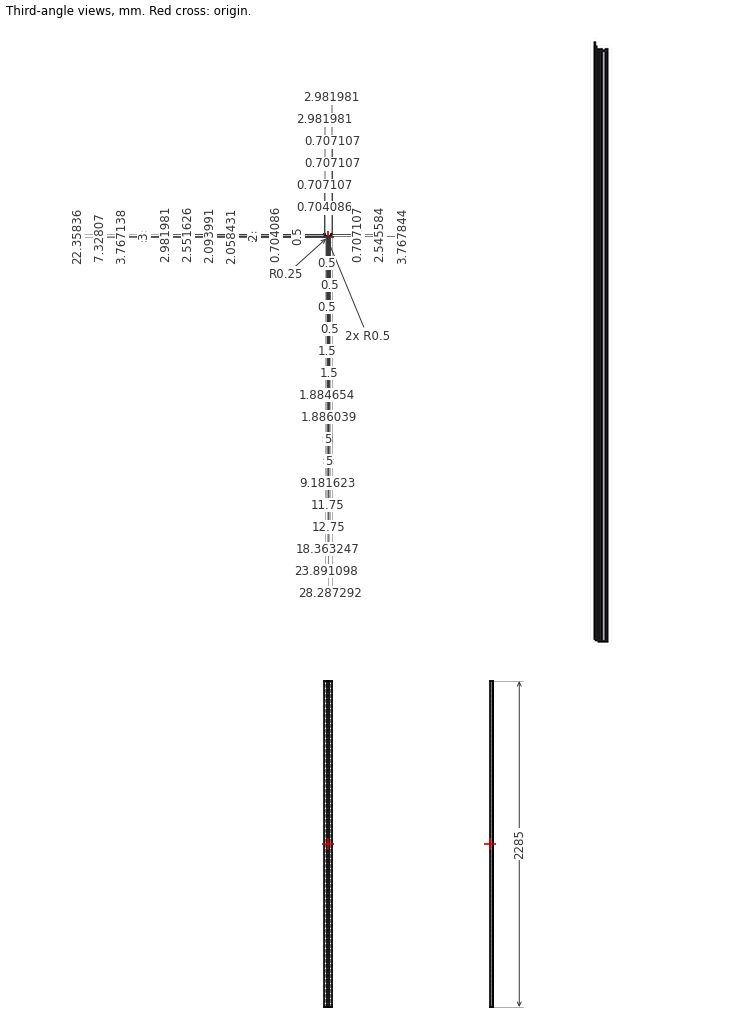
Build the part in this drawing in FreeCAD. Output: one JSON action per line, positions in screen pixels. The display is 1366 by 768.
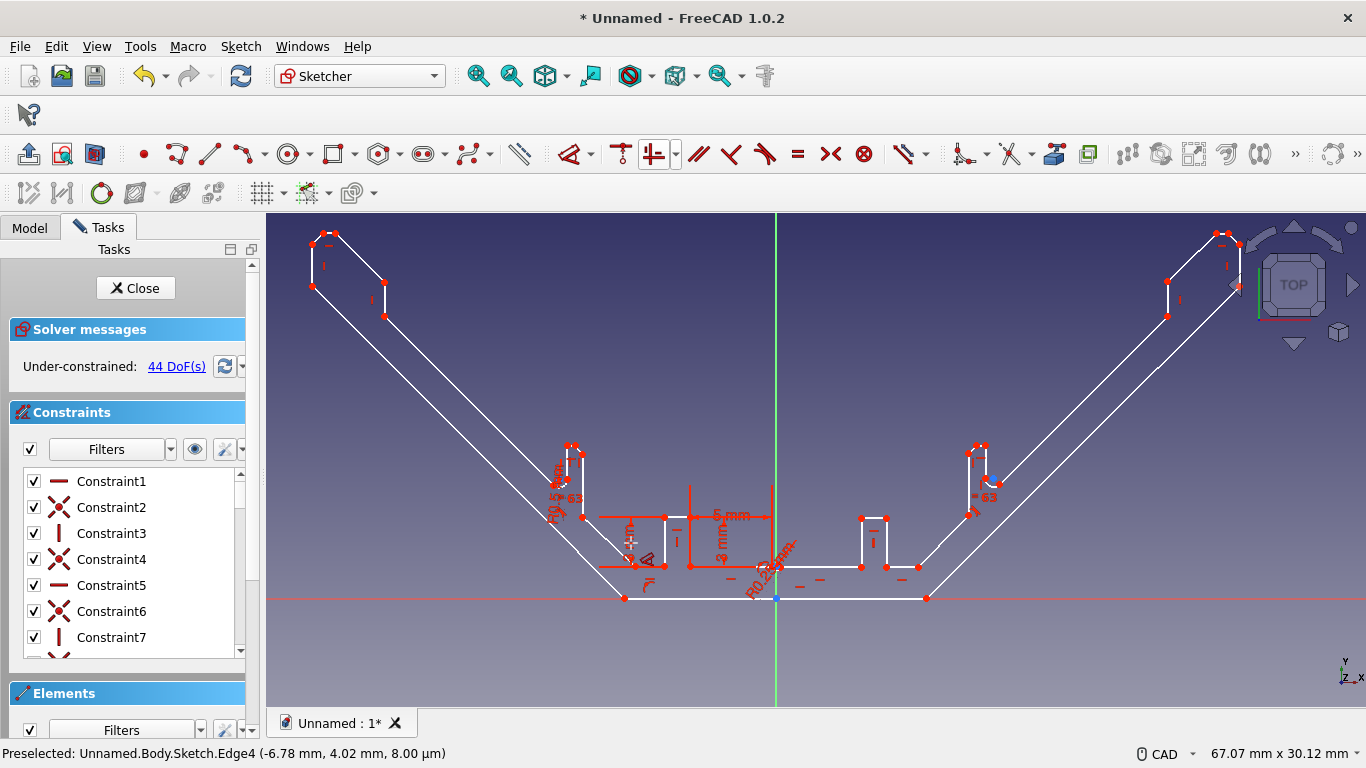
{"action": "left_click", "coordinate": [887, 552]}
{"action": "left_click", "coordinate": [921, 543]}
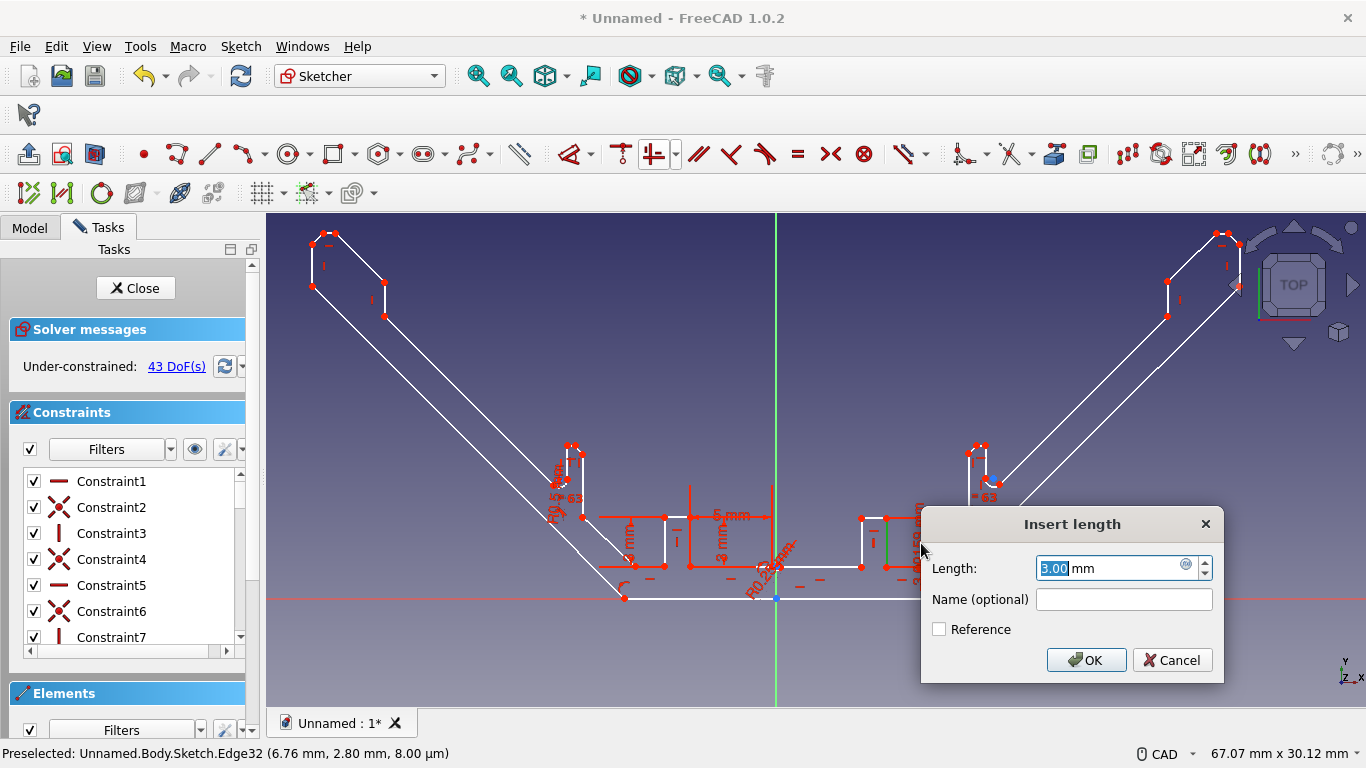
{"action": "type", "text": "3"}
{"action": "key", "text": "Return"}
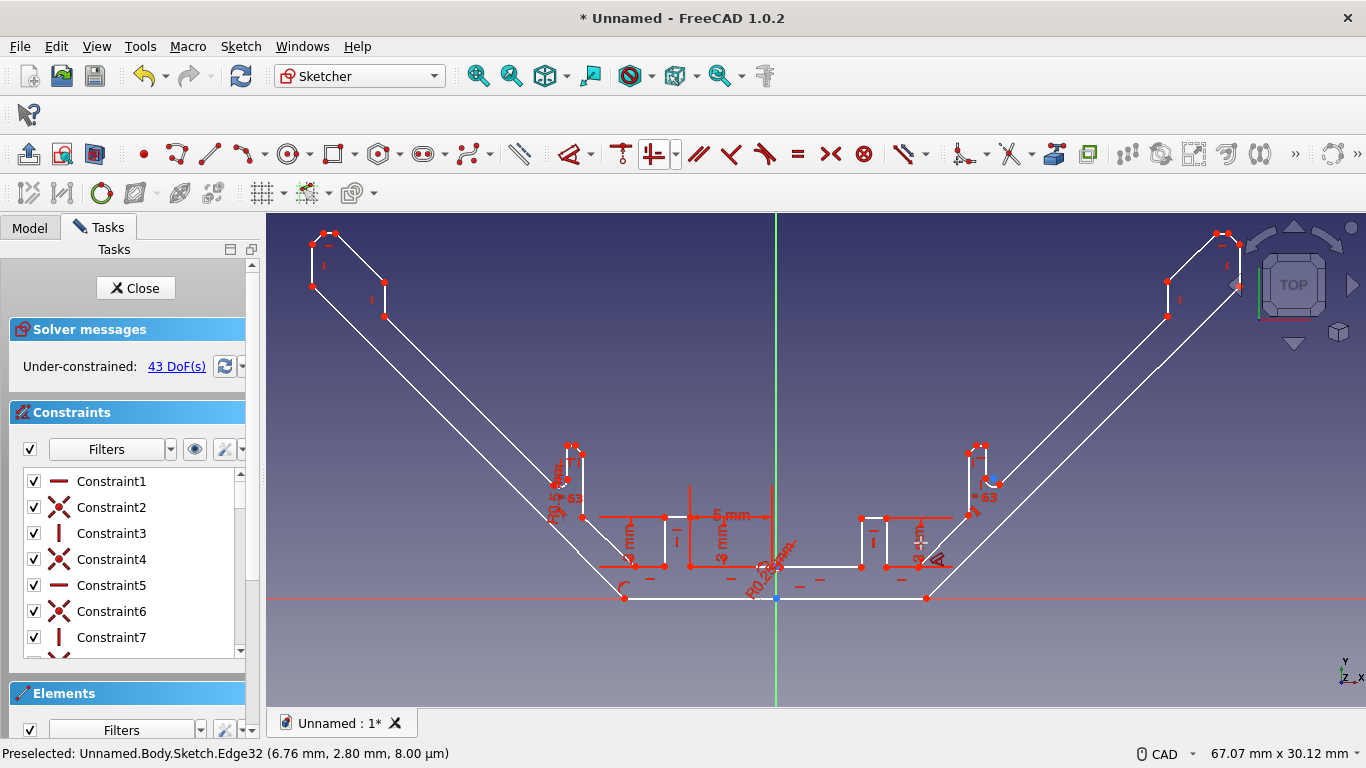
{"action": "left_click", "coordinate": [862, 533]}
{"action": "left_click", "coordinate": [828, 543]}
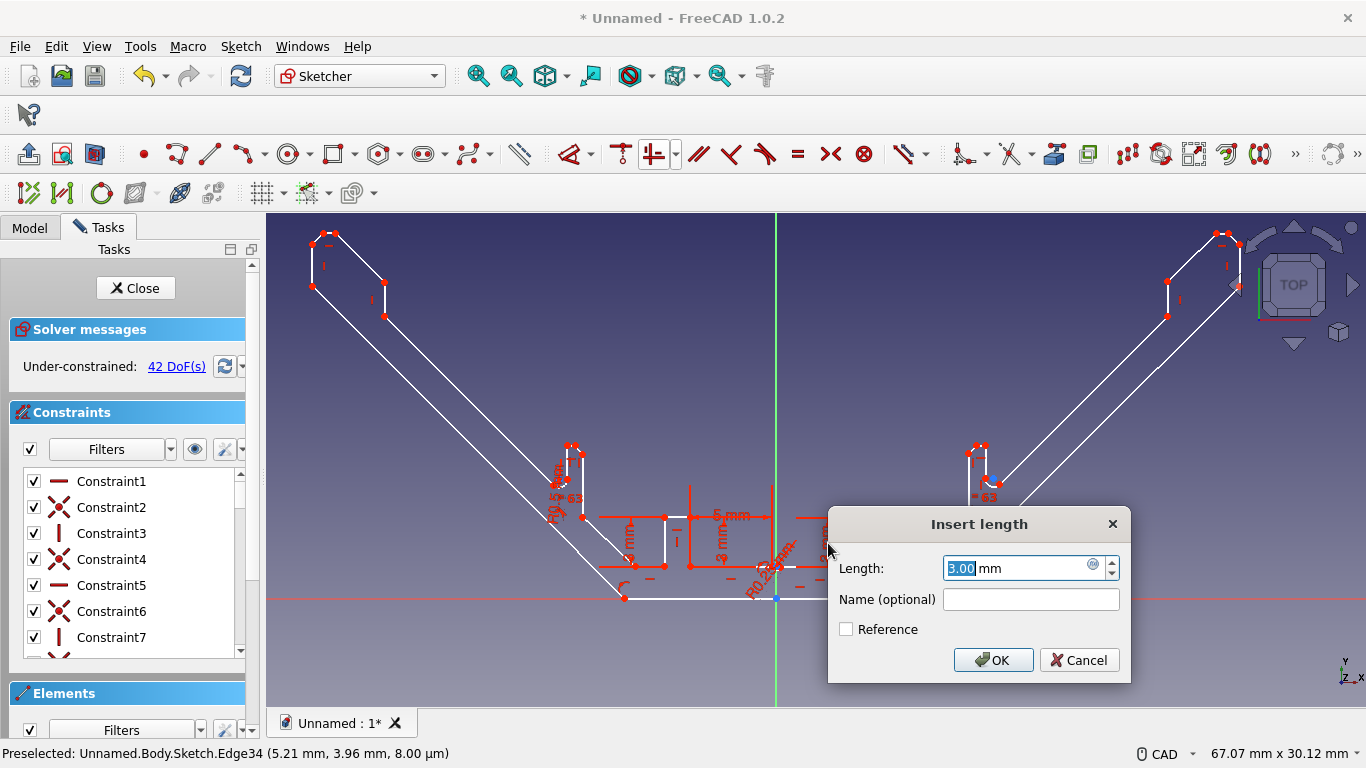
{"action": "type", "text": "3"}
{"action": "key", "text": "Return"}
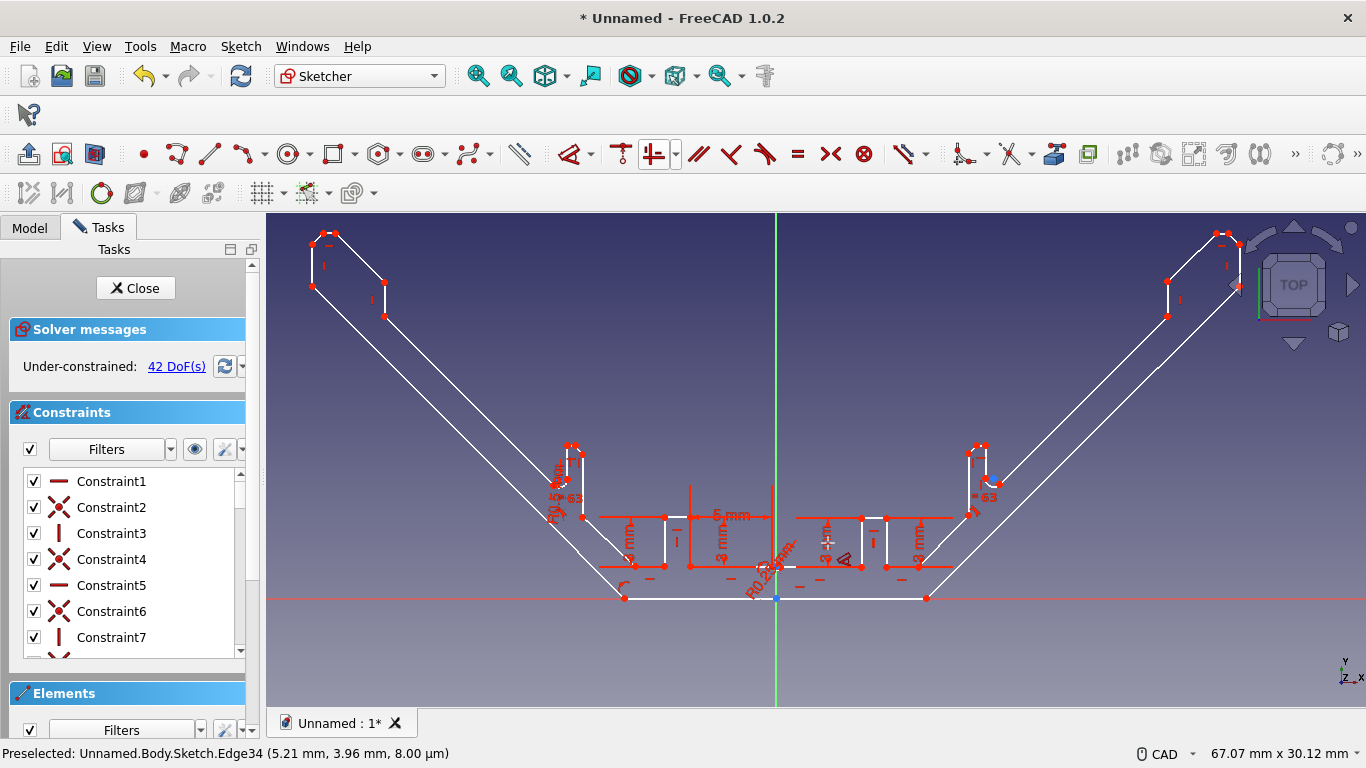
{"action": "left_click", "coordinate": [837, 567]}
{"action": "left_click", "coordinate": [821, 625]}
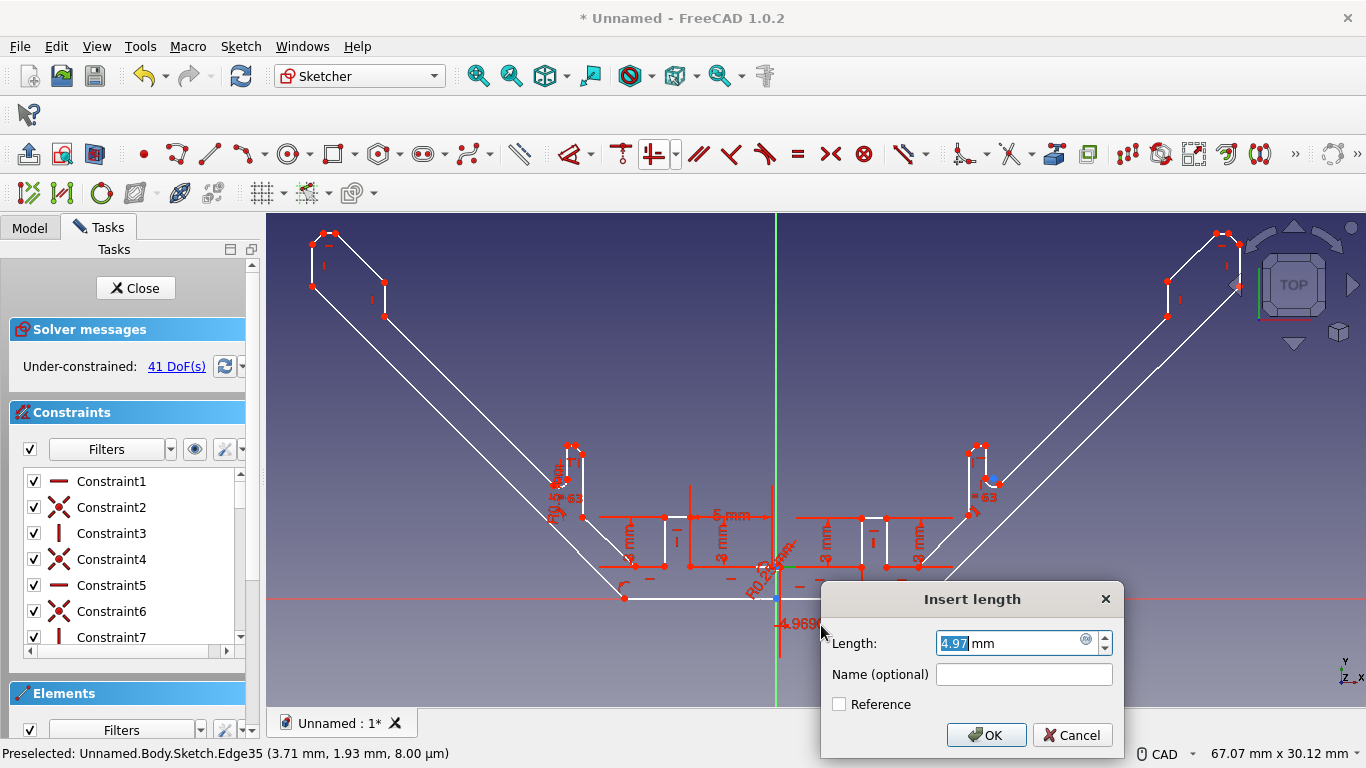
{"action": "type", "text": "5"}
{"action": "key", "text": "Return"}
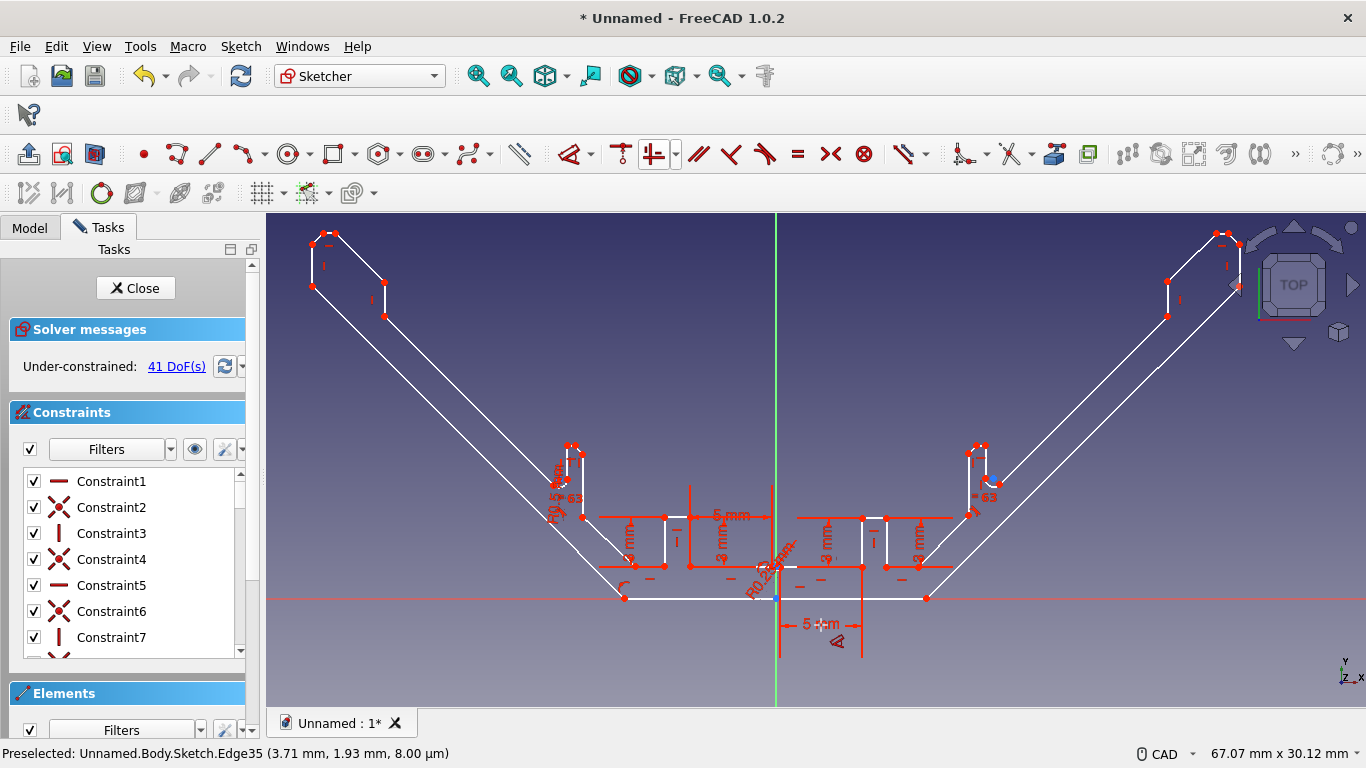
{"action": "scroll", "coordinate": [772, 567], "scroll_direction": "up", "scroll_amount": 6}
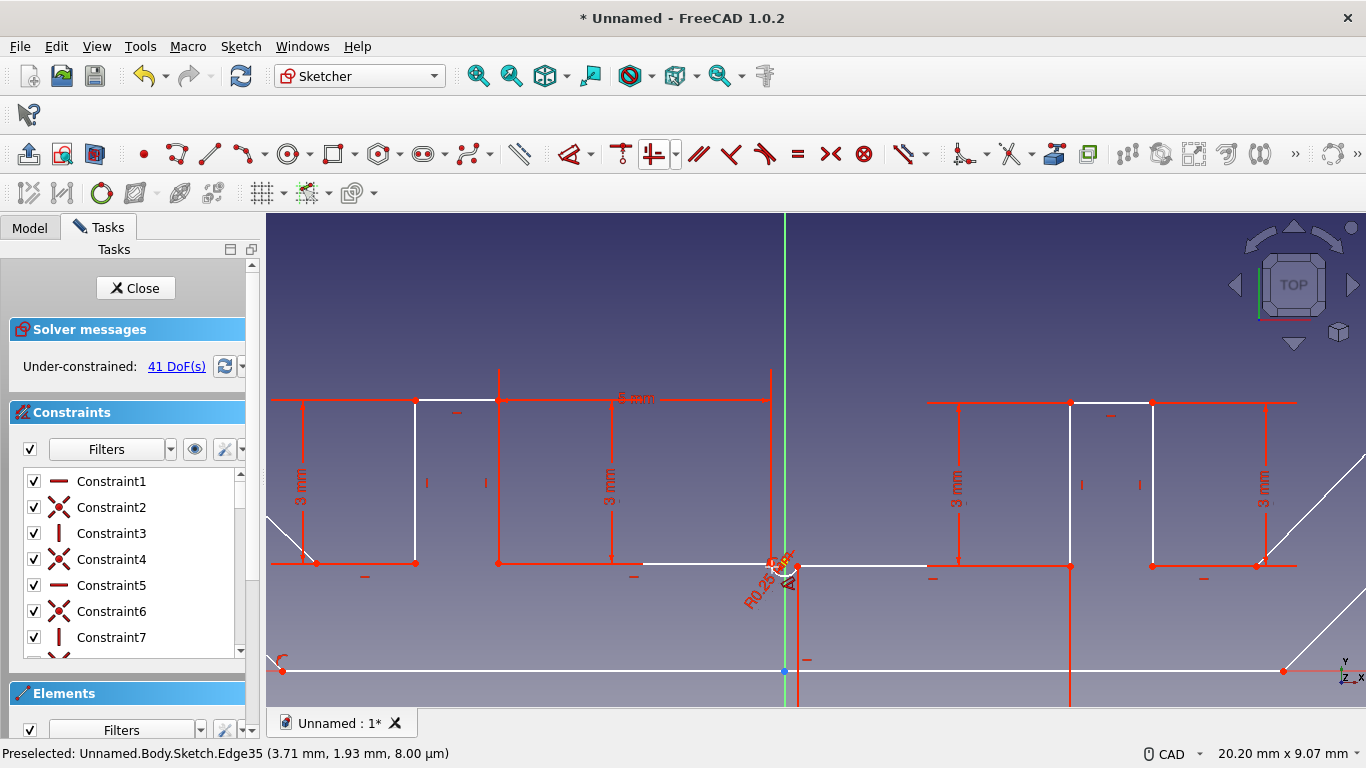
{"action": "left_click", "coordinate": [771, 564]}
{"action": "left_click", "coordinate": [737, 618]}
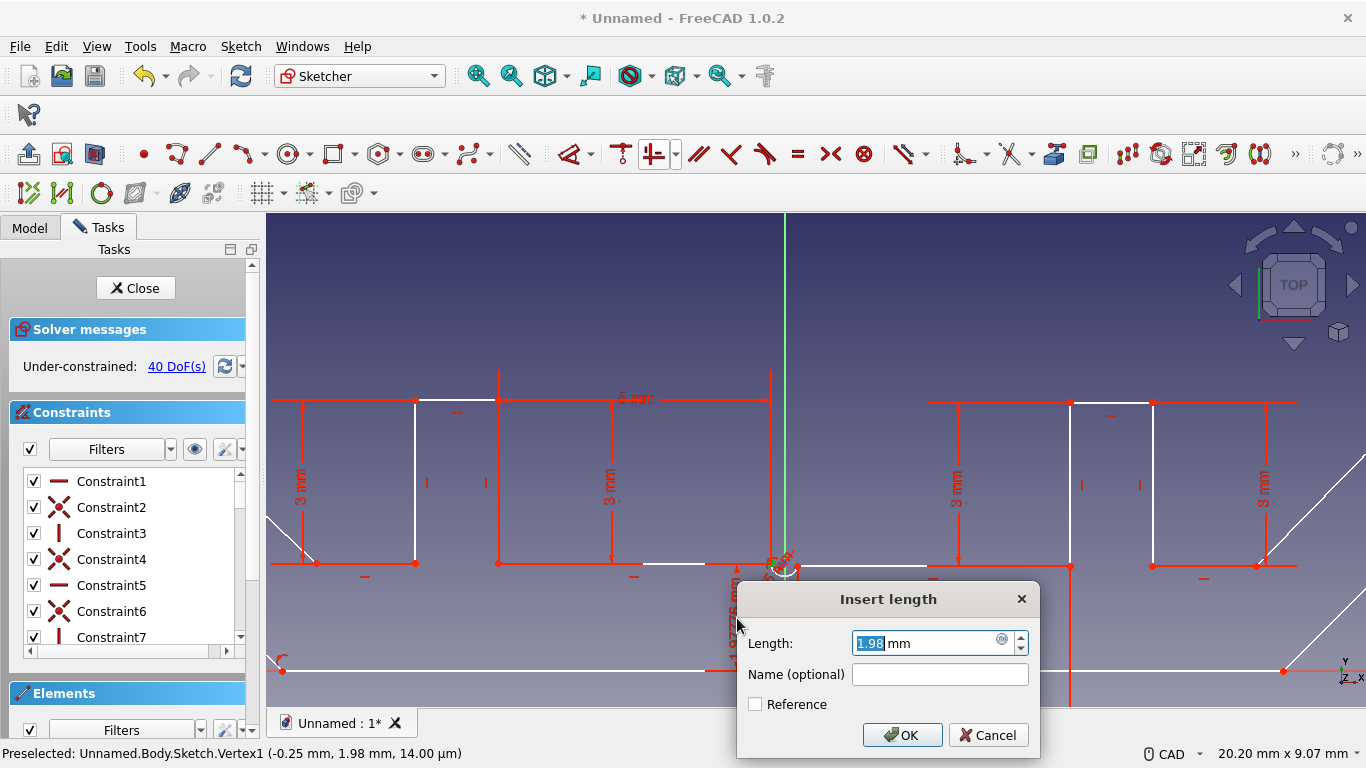
{"action": "type", "text": "2"}
{"action": "key", "text": "Return"}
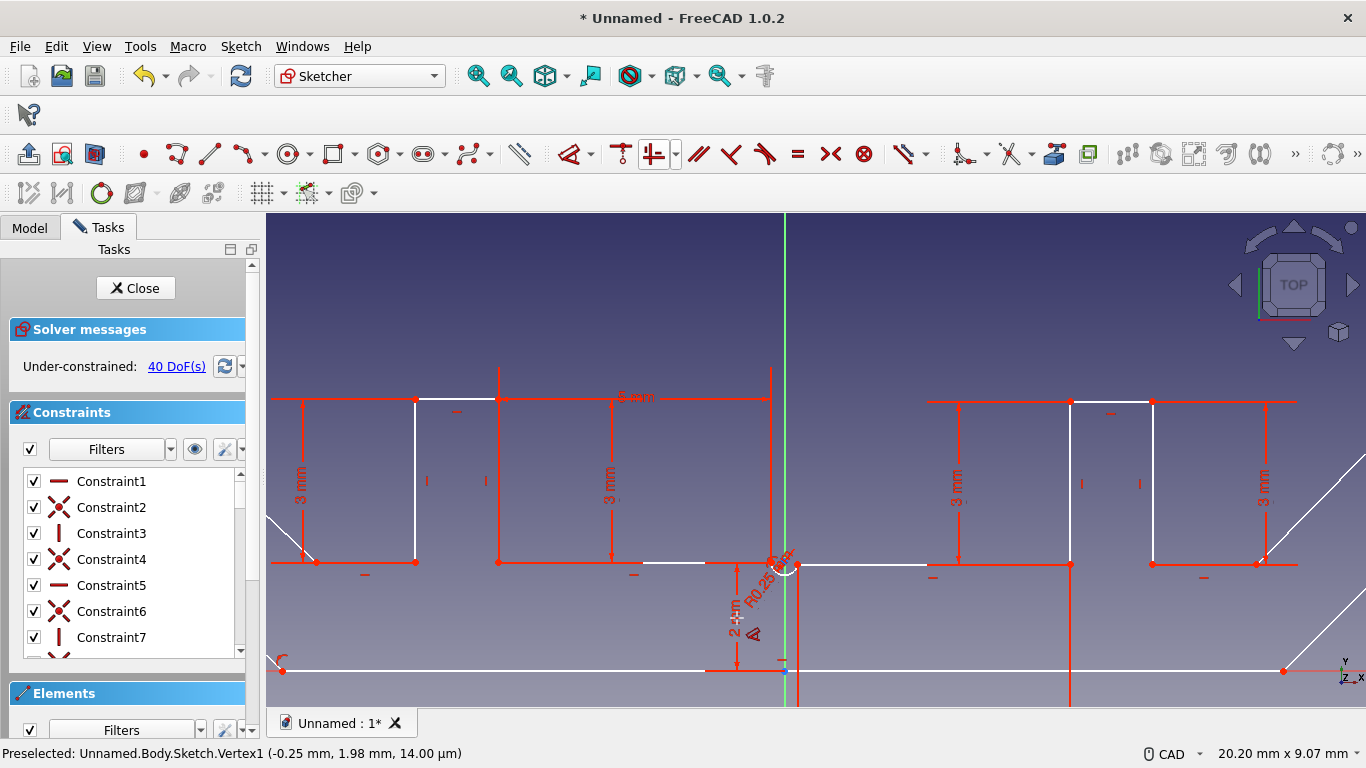
{"action": "scroll", "coordinate": [738, 560], "scroll_direction": "down", "scroll_amount": 8}